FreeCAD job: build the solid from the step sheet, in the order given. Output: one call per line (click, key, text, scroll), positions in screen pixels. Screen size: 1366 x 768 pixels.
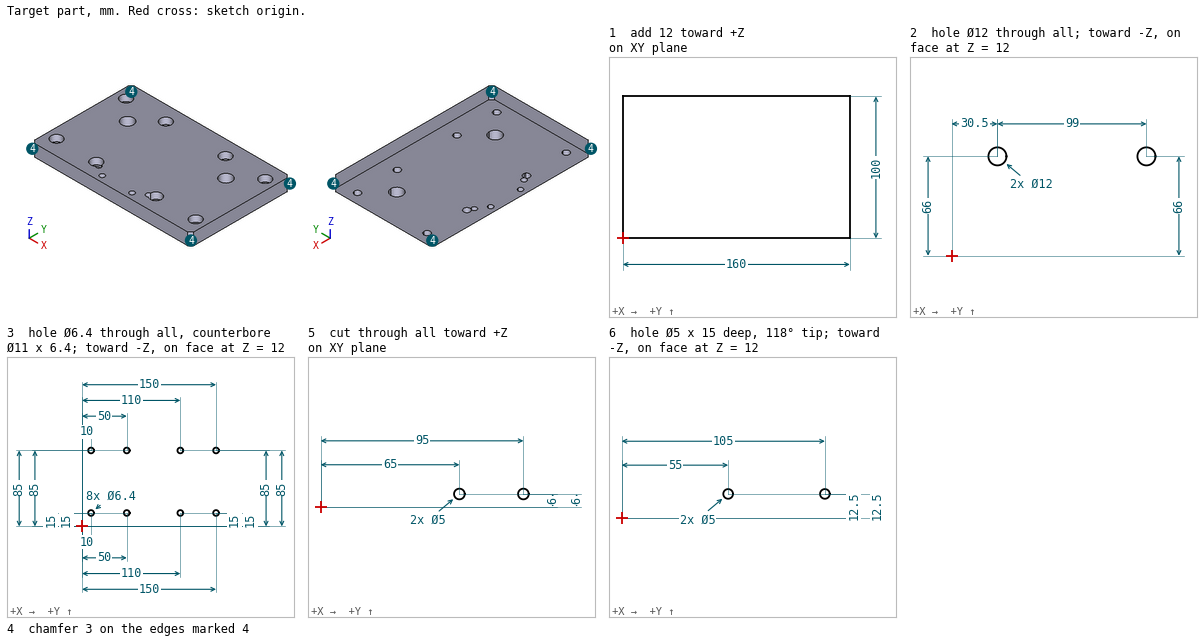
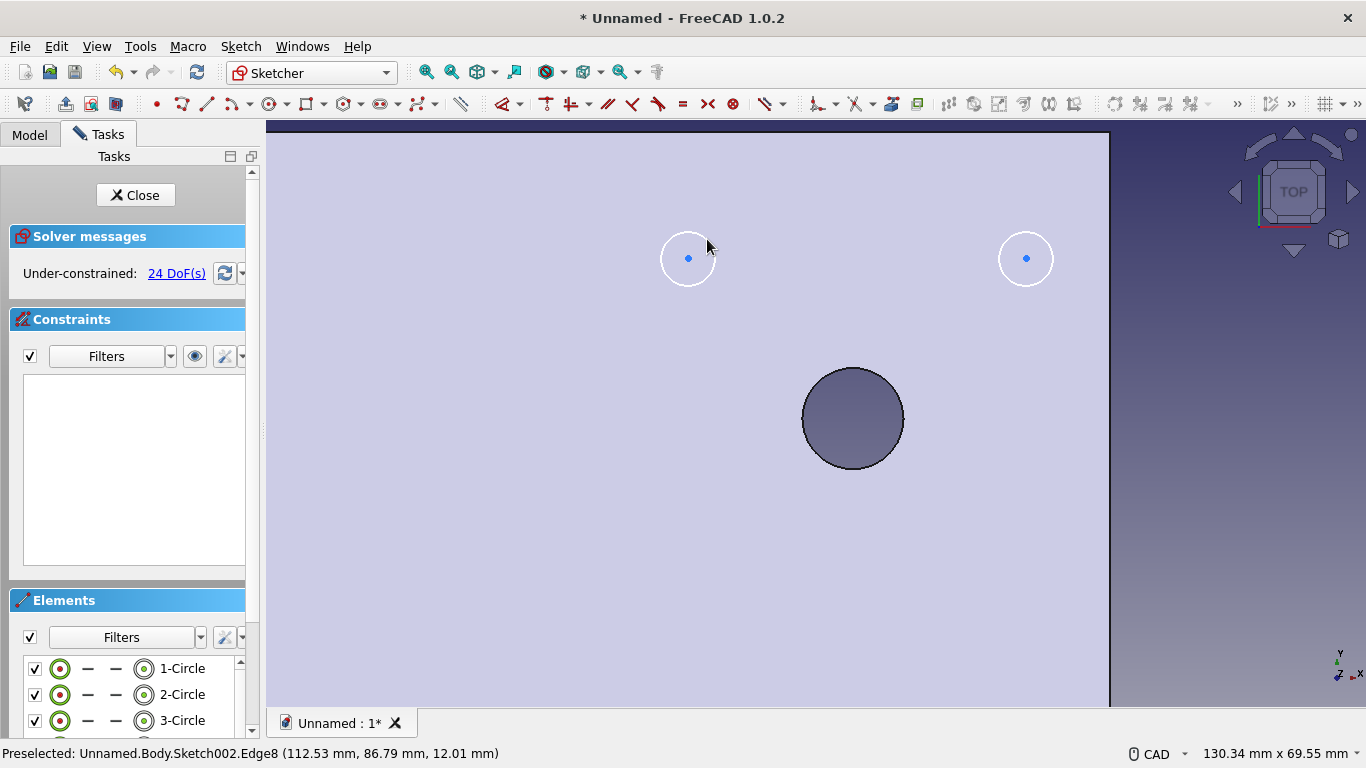
scroll(1026, 258, down, 4)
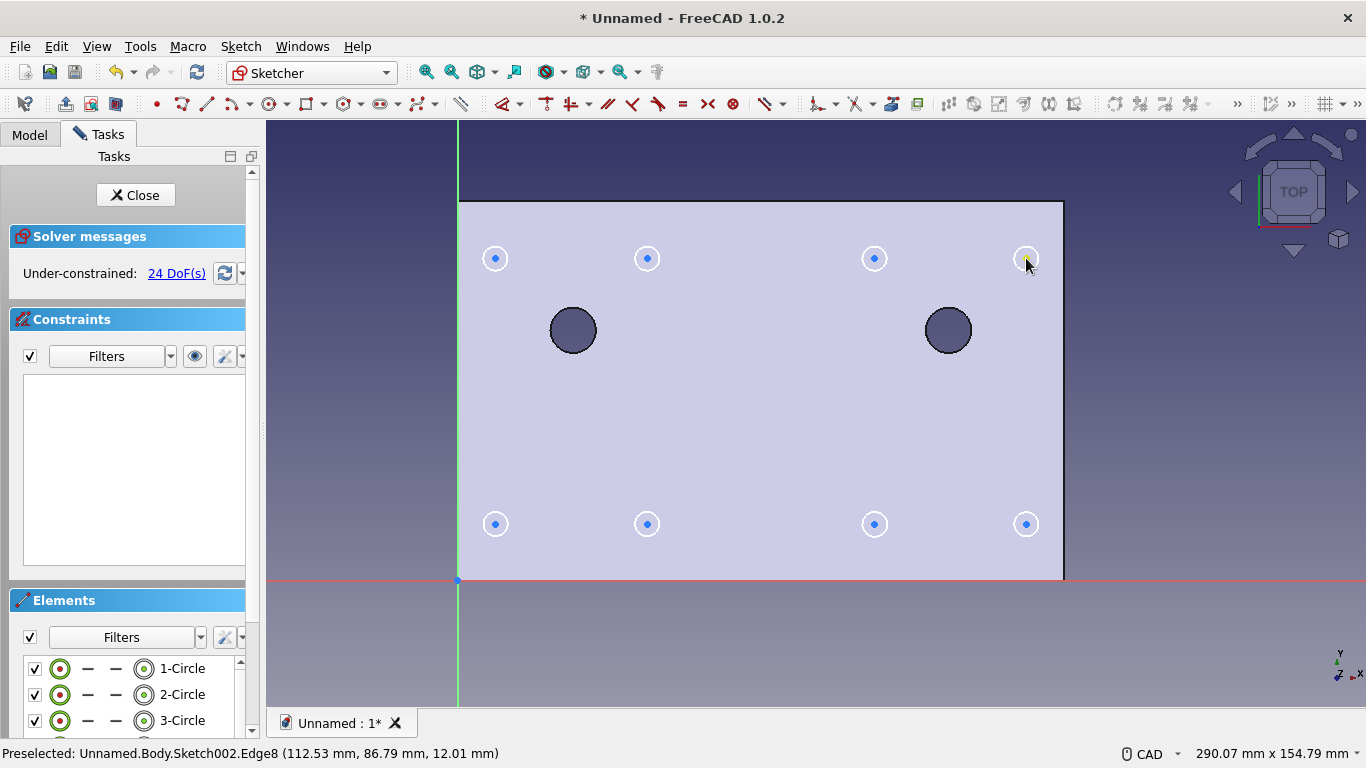
click(504, 515)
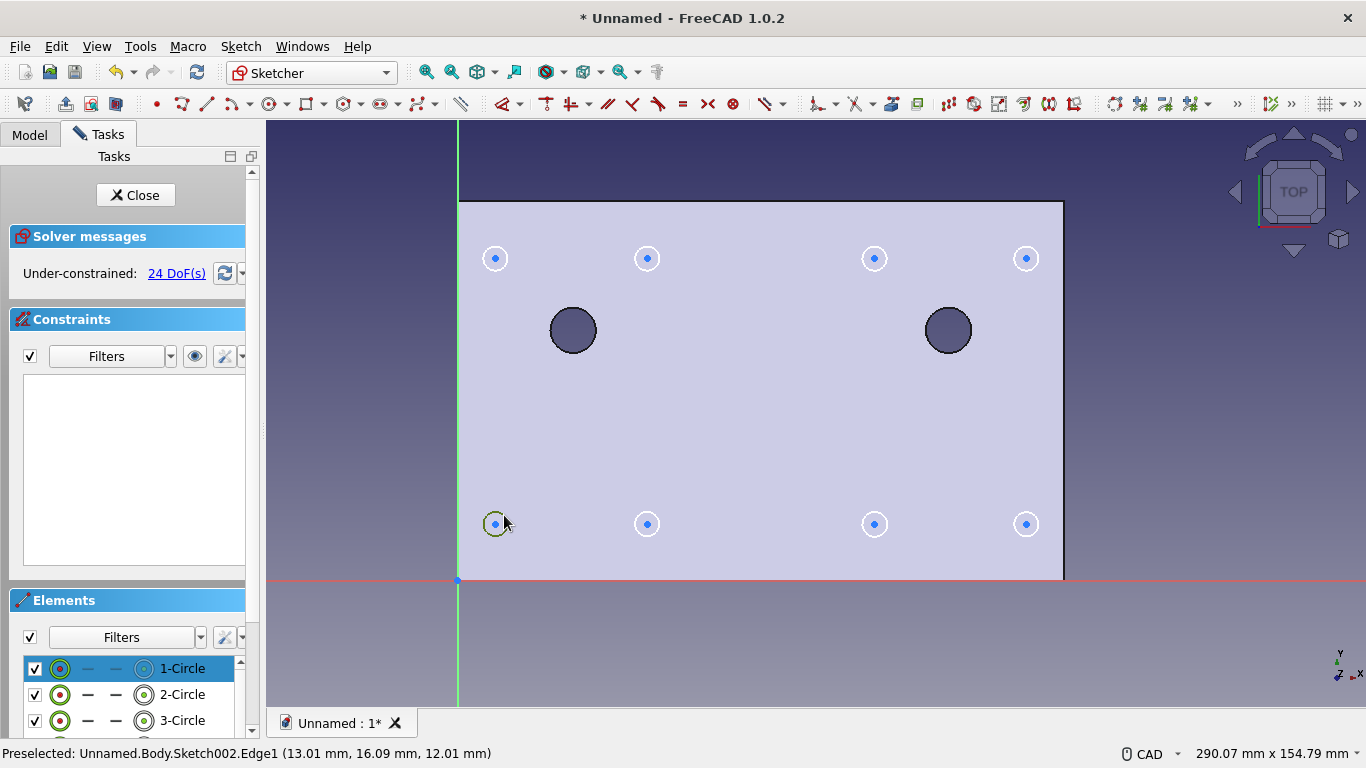
click(656, 515)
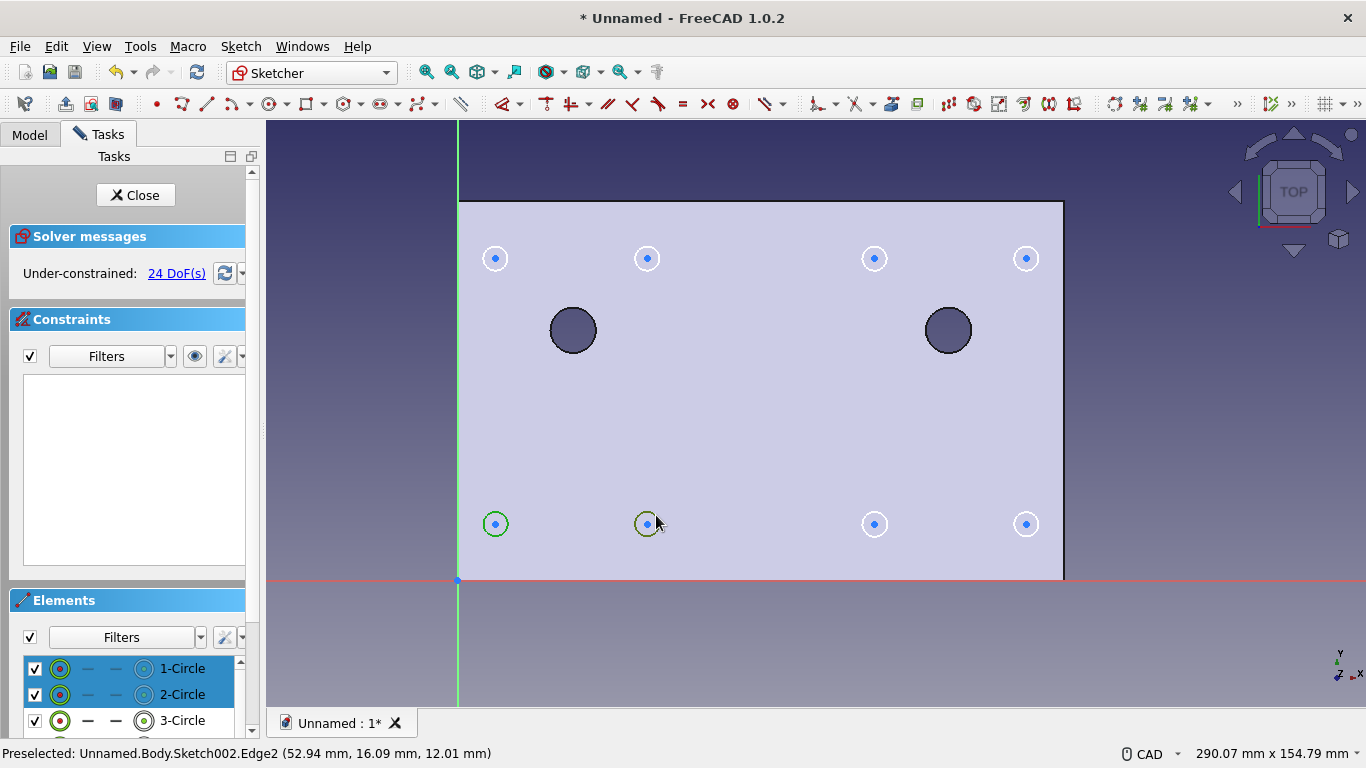
click(656, 250)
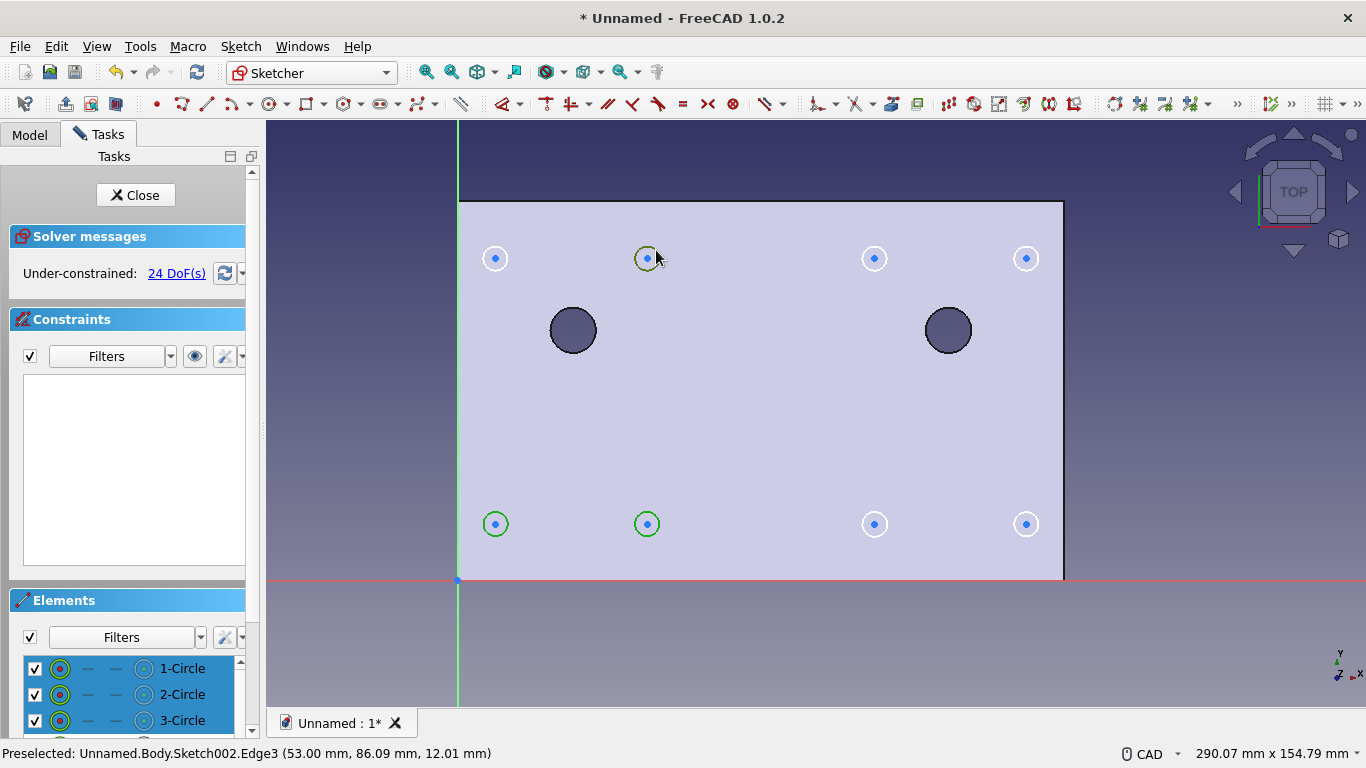
click(504, 250)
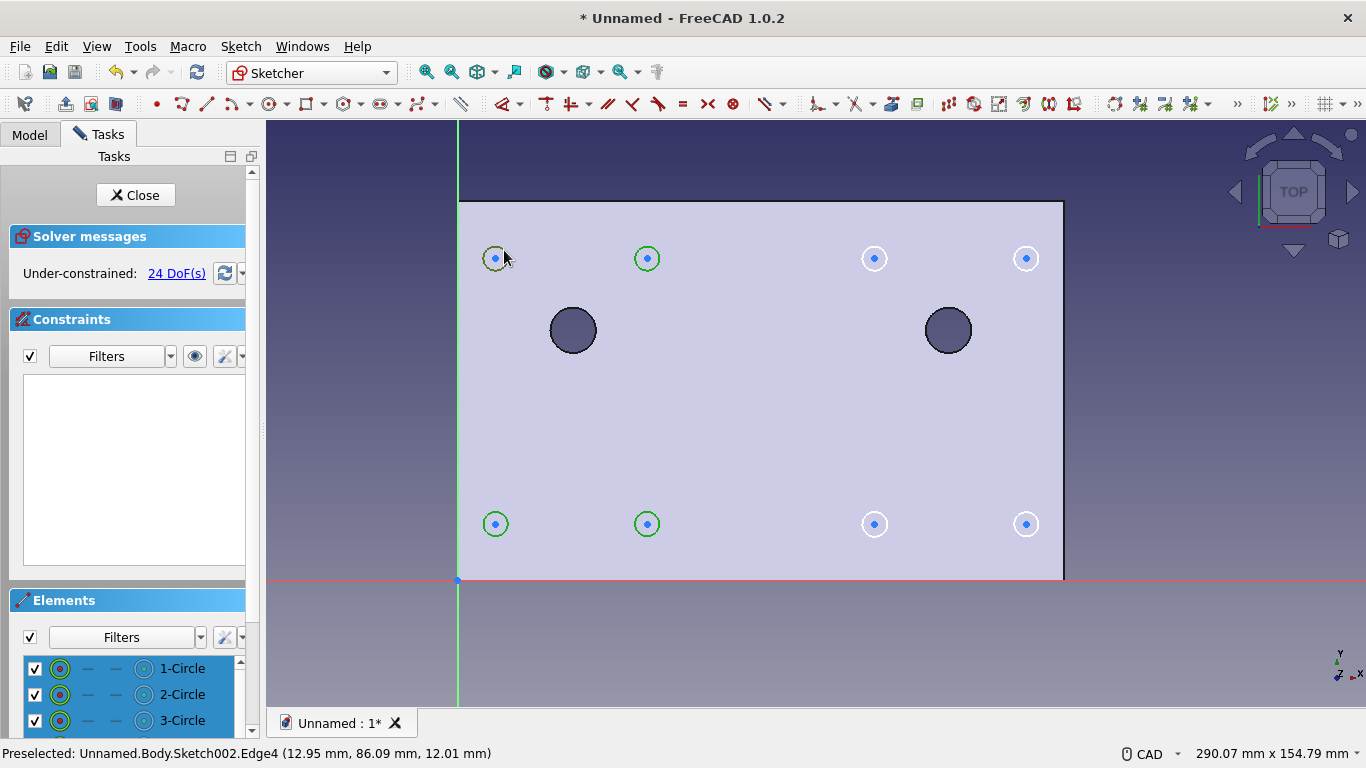
click(884, 516)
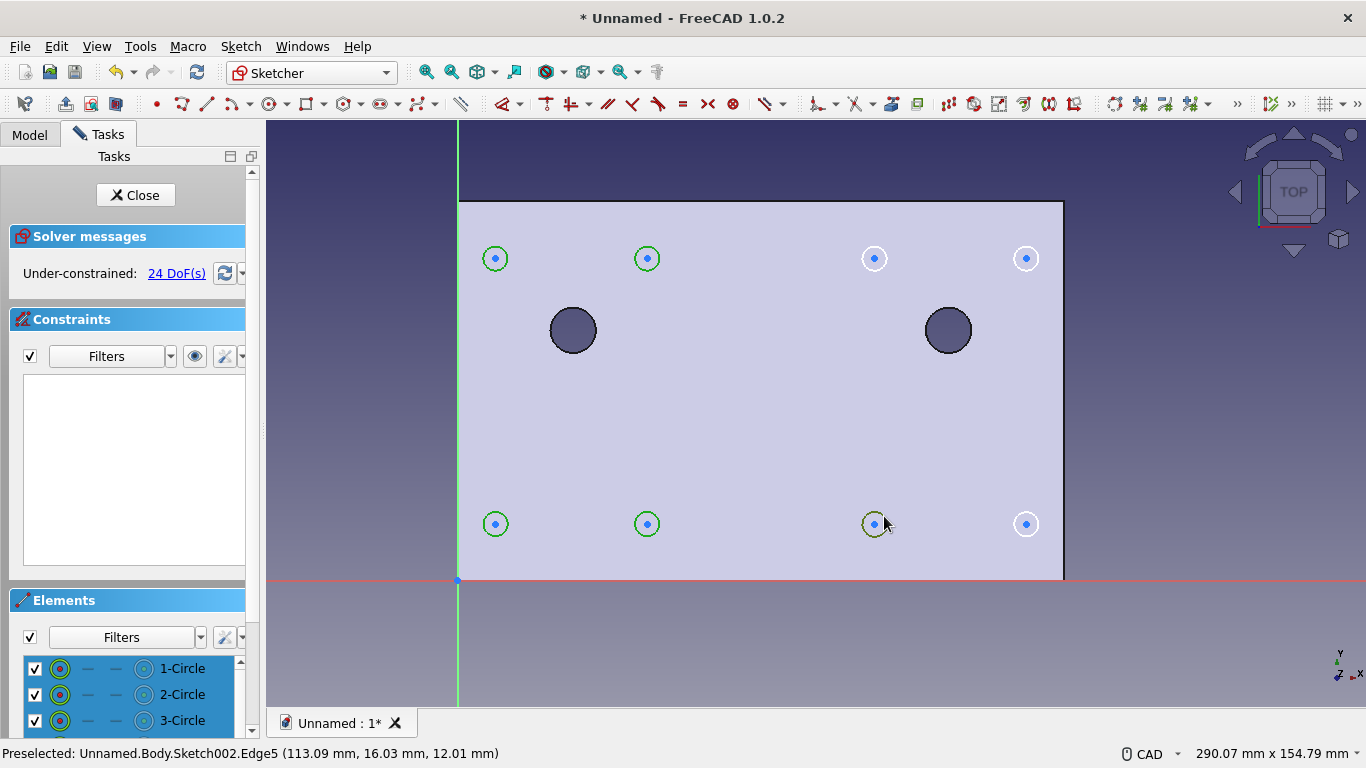
click(1035, 516)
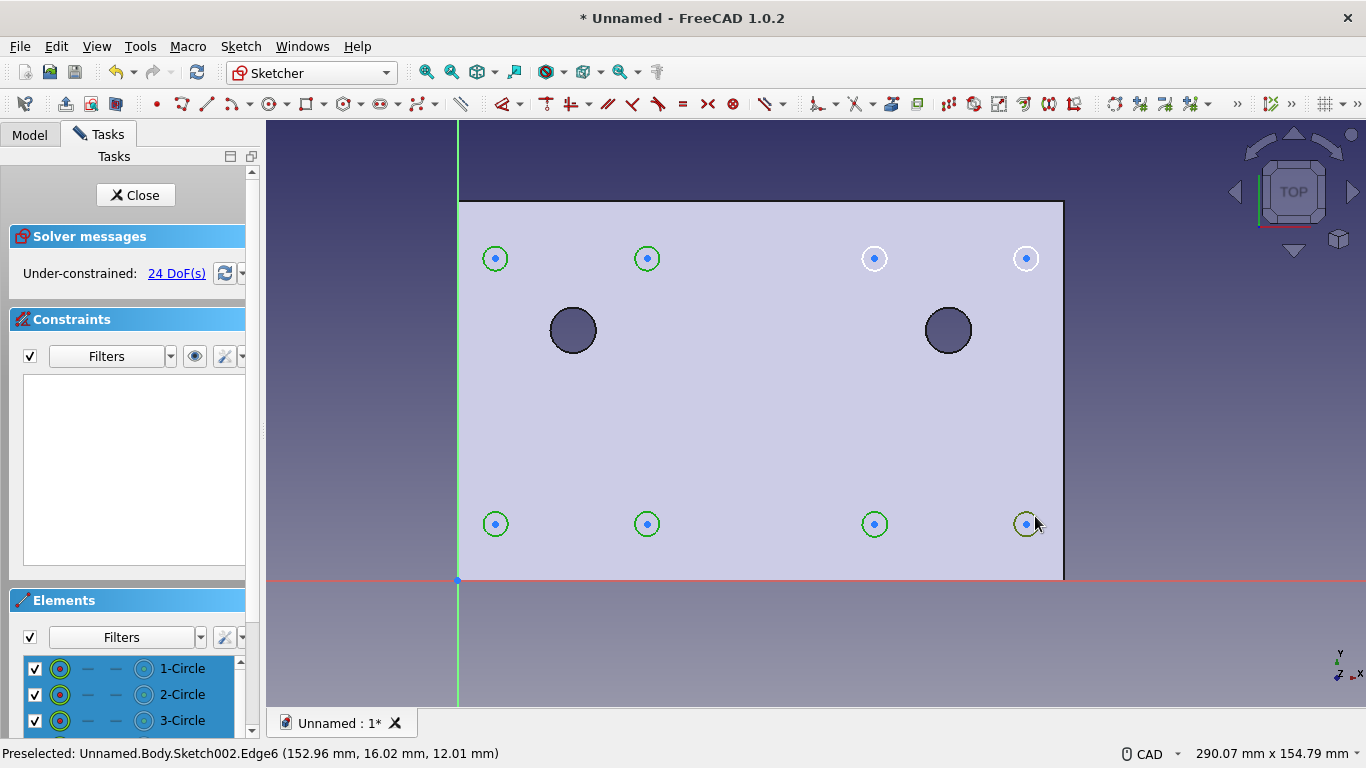
click(1035, 250)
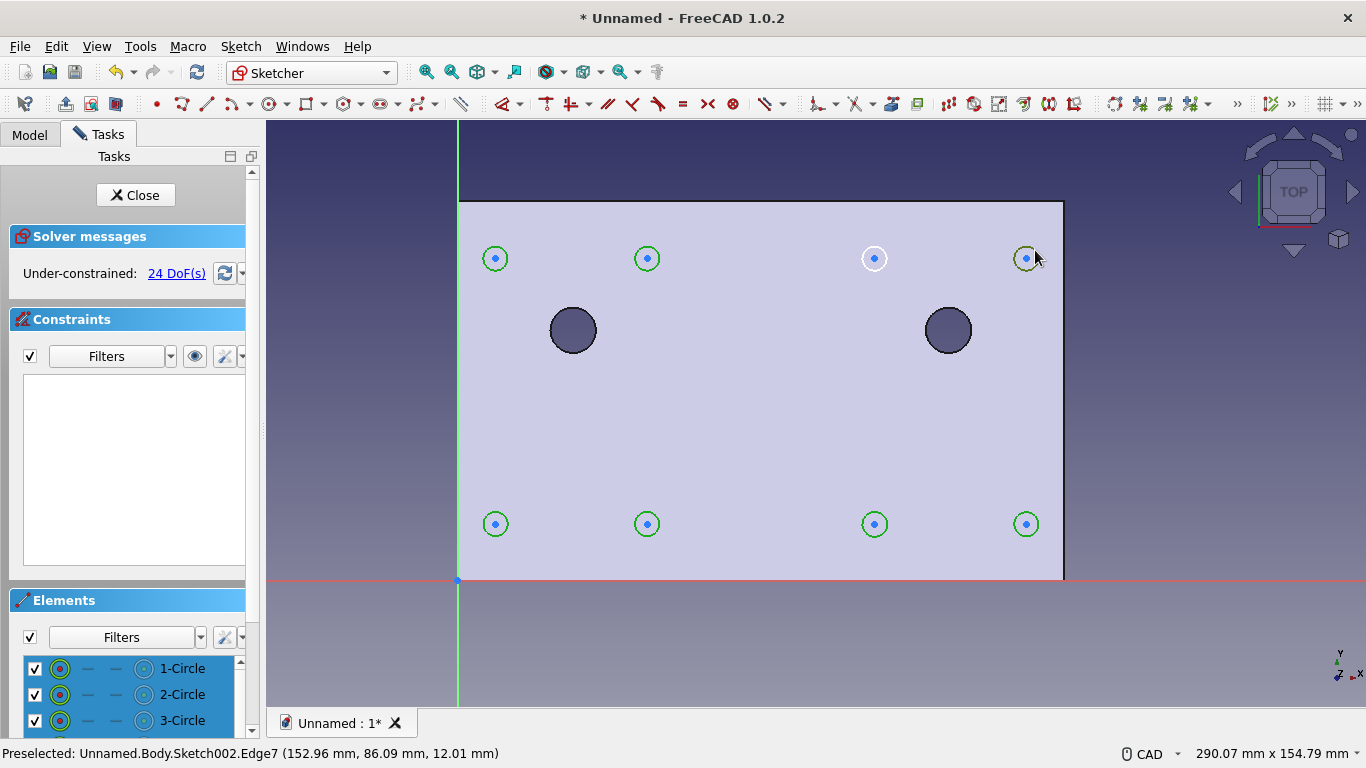
click(883, 250)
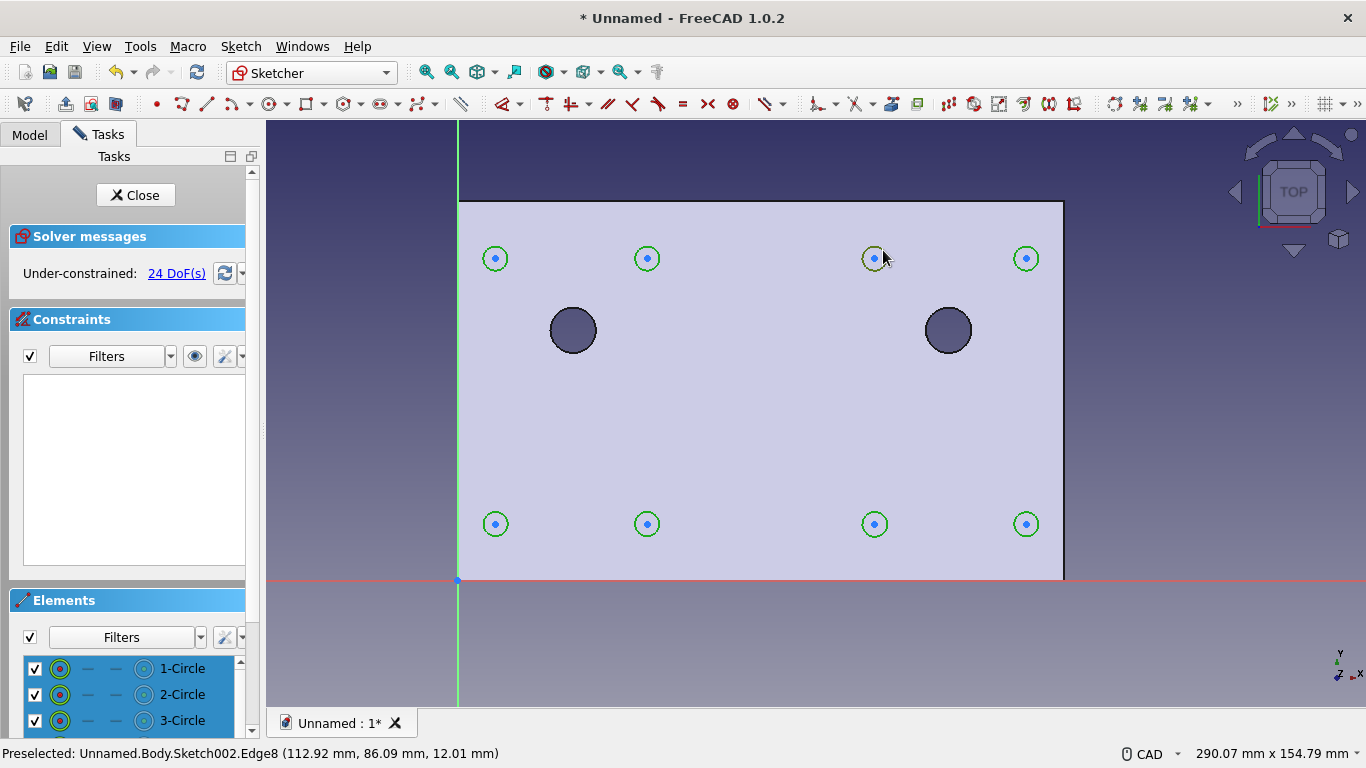
key(e)